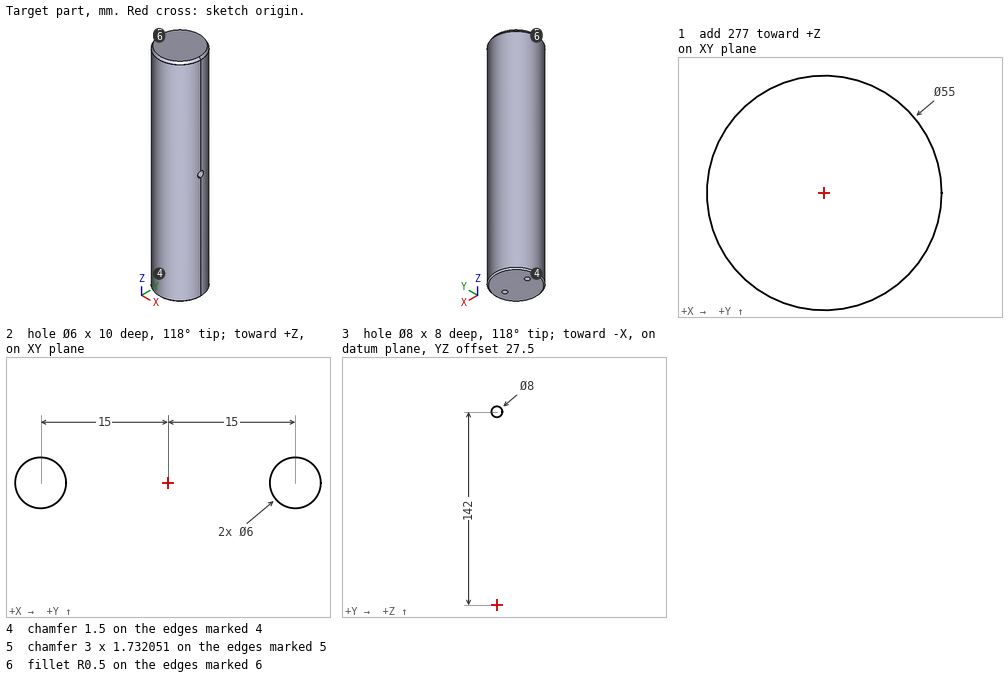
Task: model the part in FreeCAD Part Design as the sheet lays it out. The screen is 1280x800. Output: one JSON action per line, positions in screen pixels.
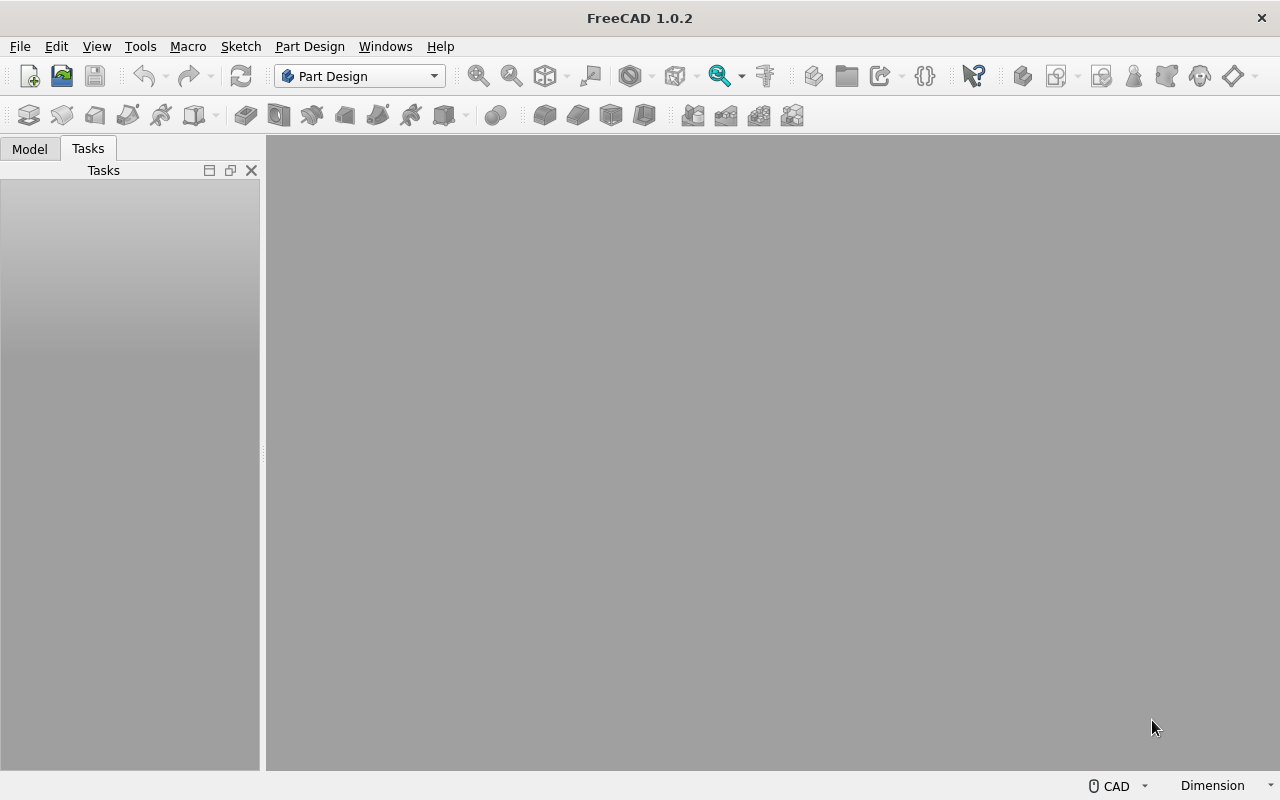
{"action": "left_click", "coordinate": [29, 76]}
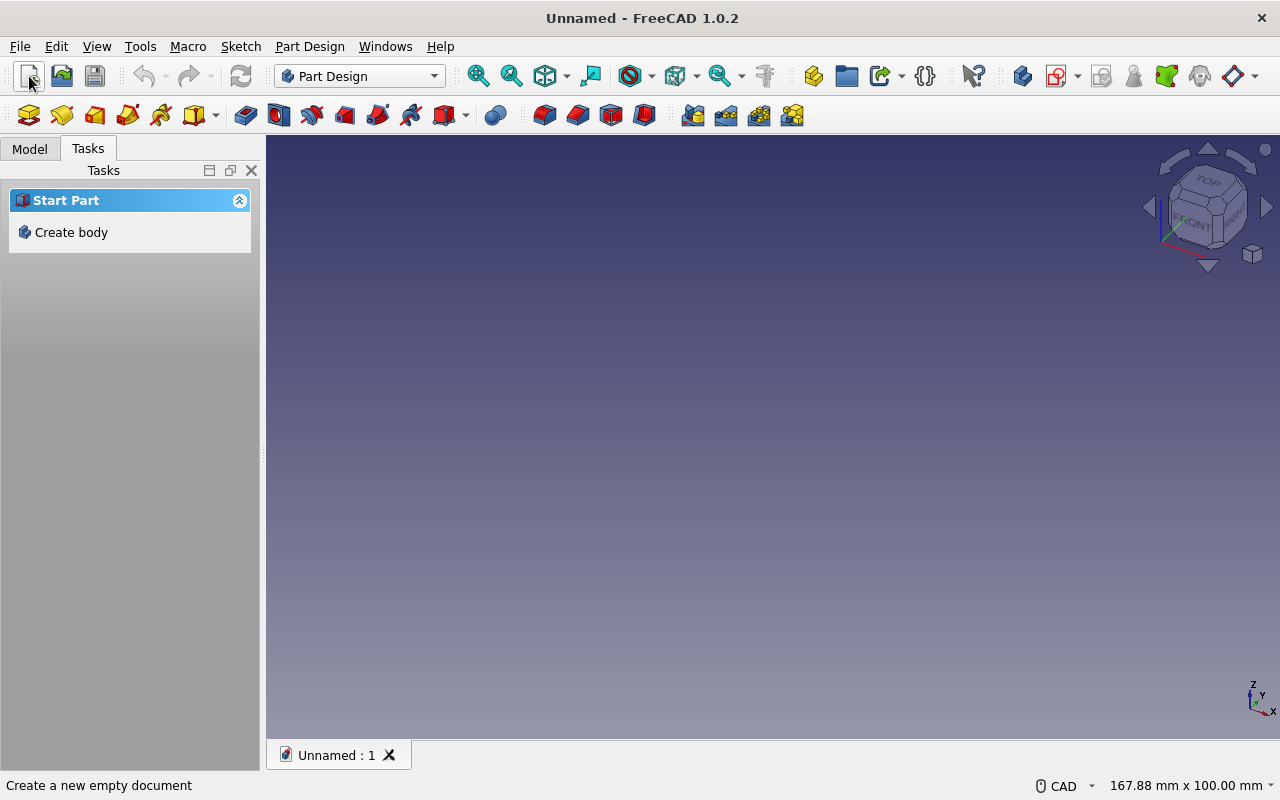
{"action": "left_click", "coordinate": [1056, 76]}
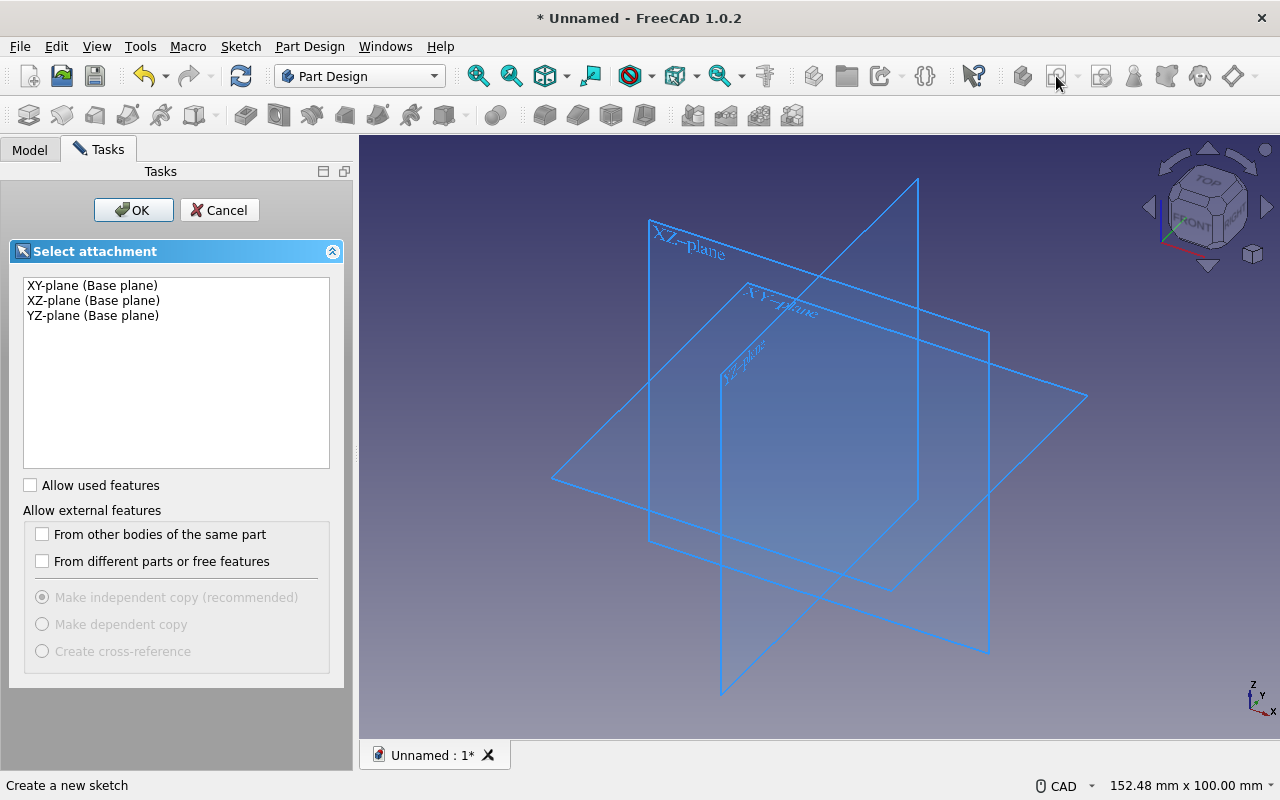
{"action": "left_click", "coordinate": [84, 286]}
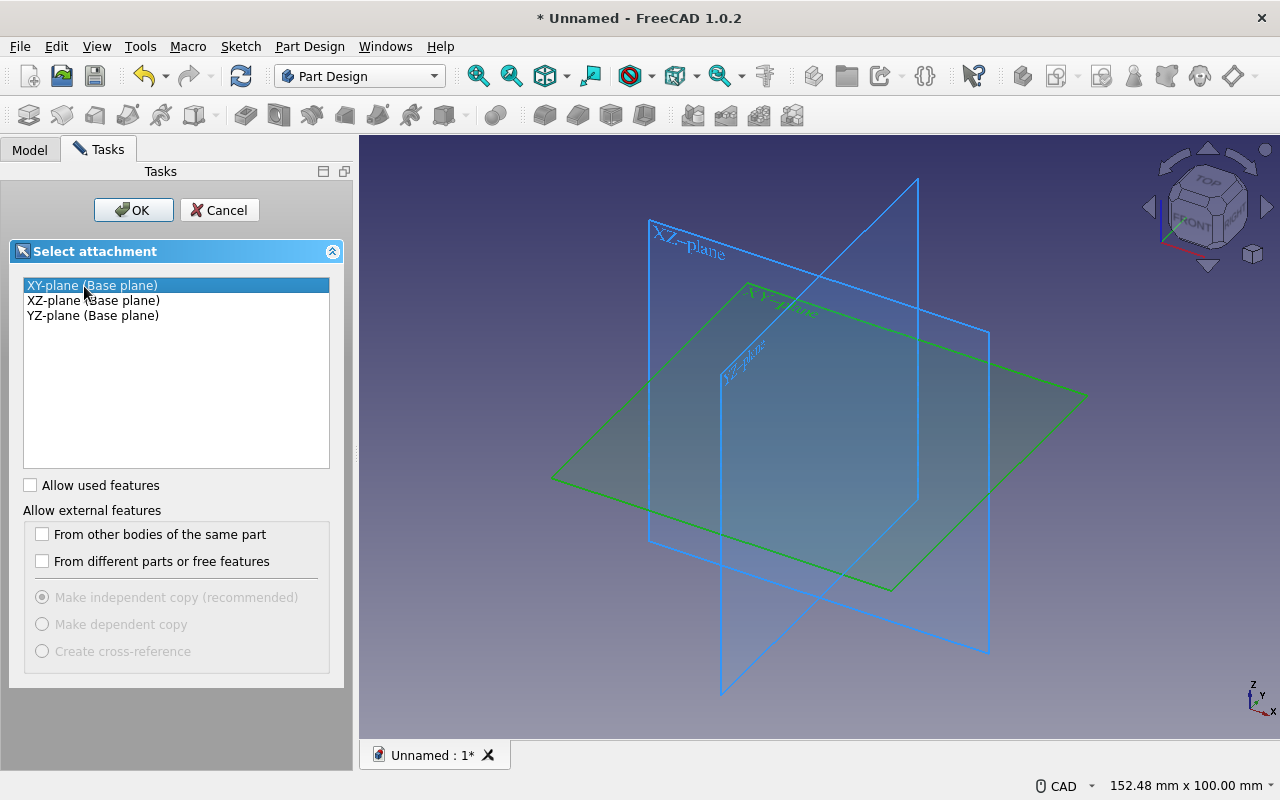
{"action": "left_click", "coordinate": [134, 210]}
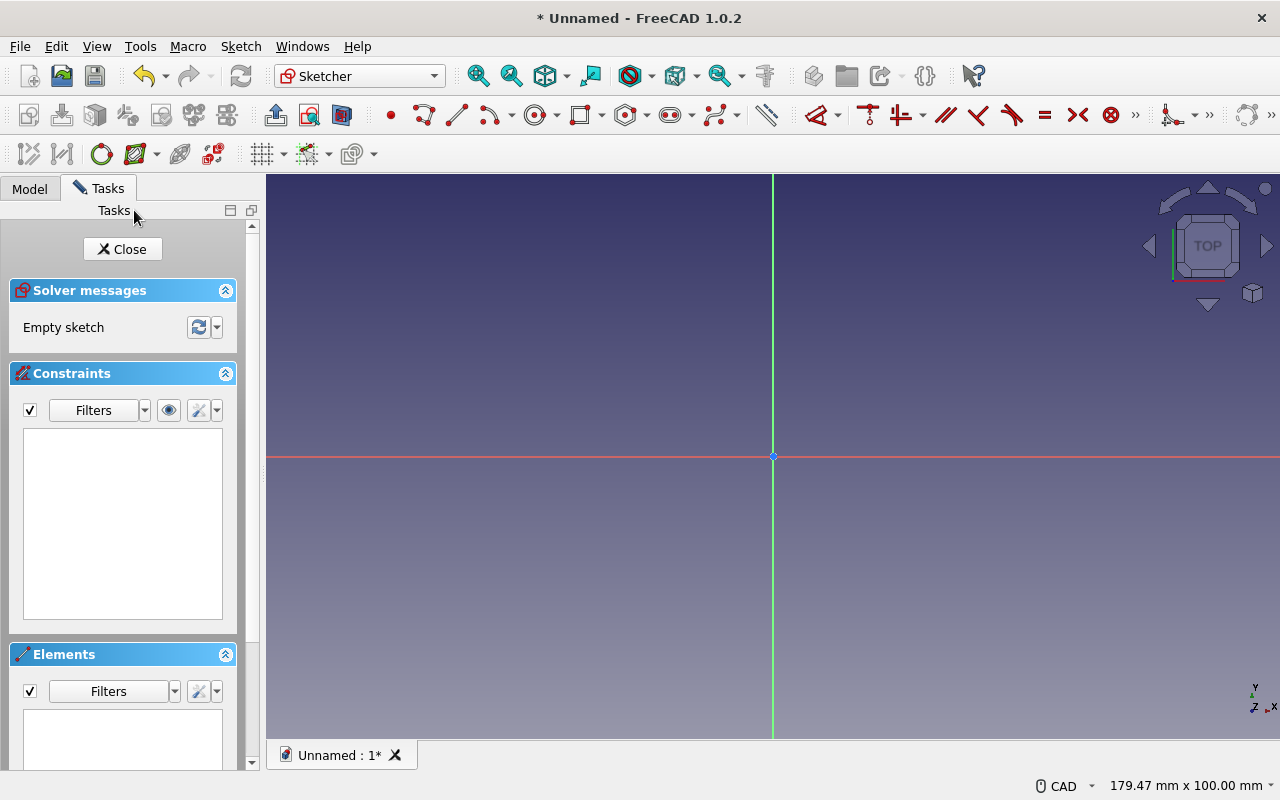
{"action": "left_click", "coordinate": [534, 116]}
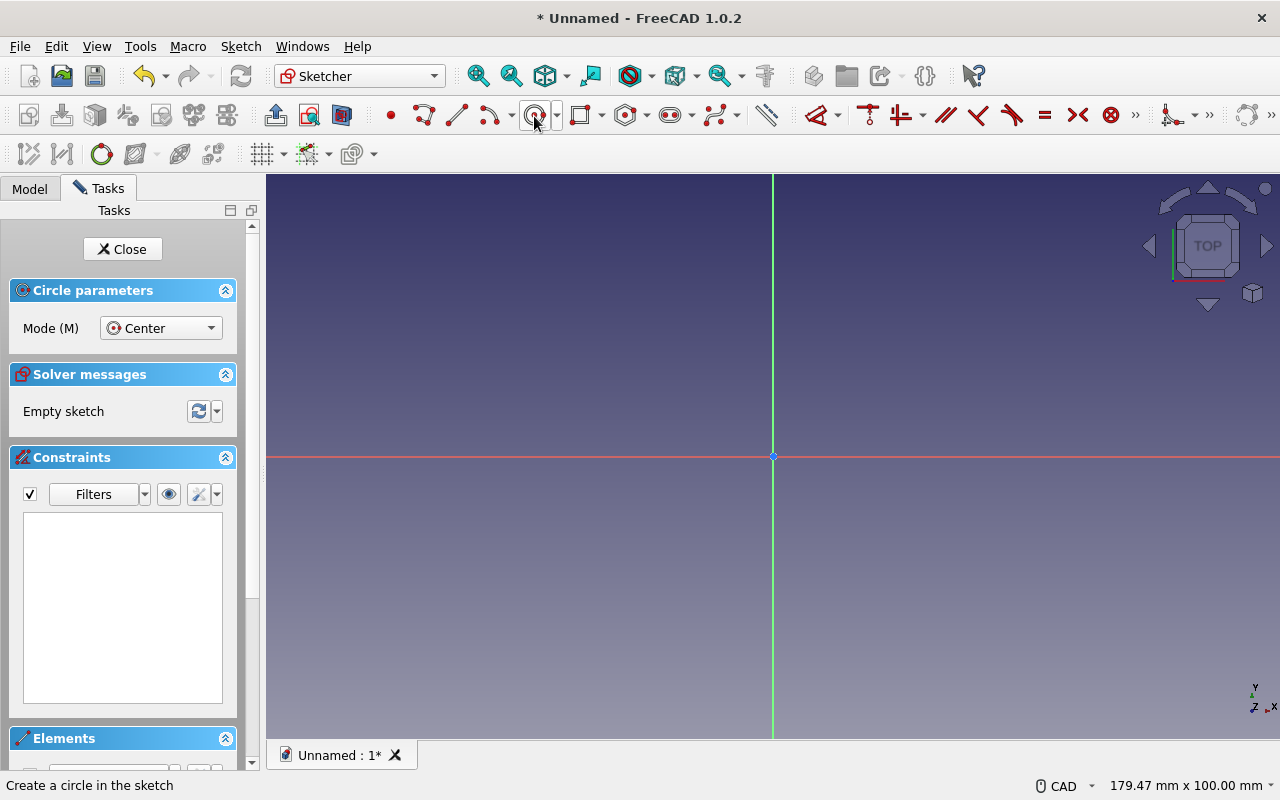
{"action": "left_click", "coordinate": [773, 456]}
{"action": "left_click", "coordinate": [883, 347]}
{"action": "key", "text": "Escape"}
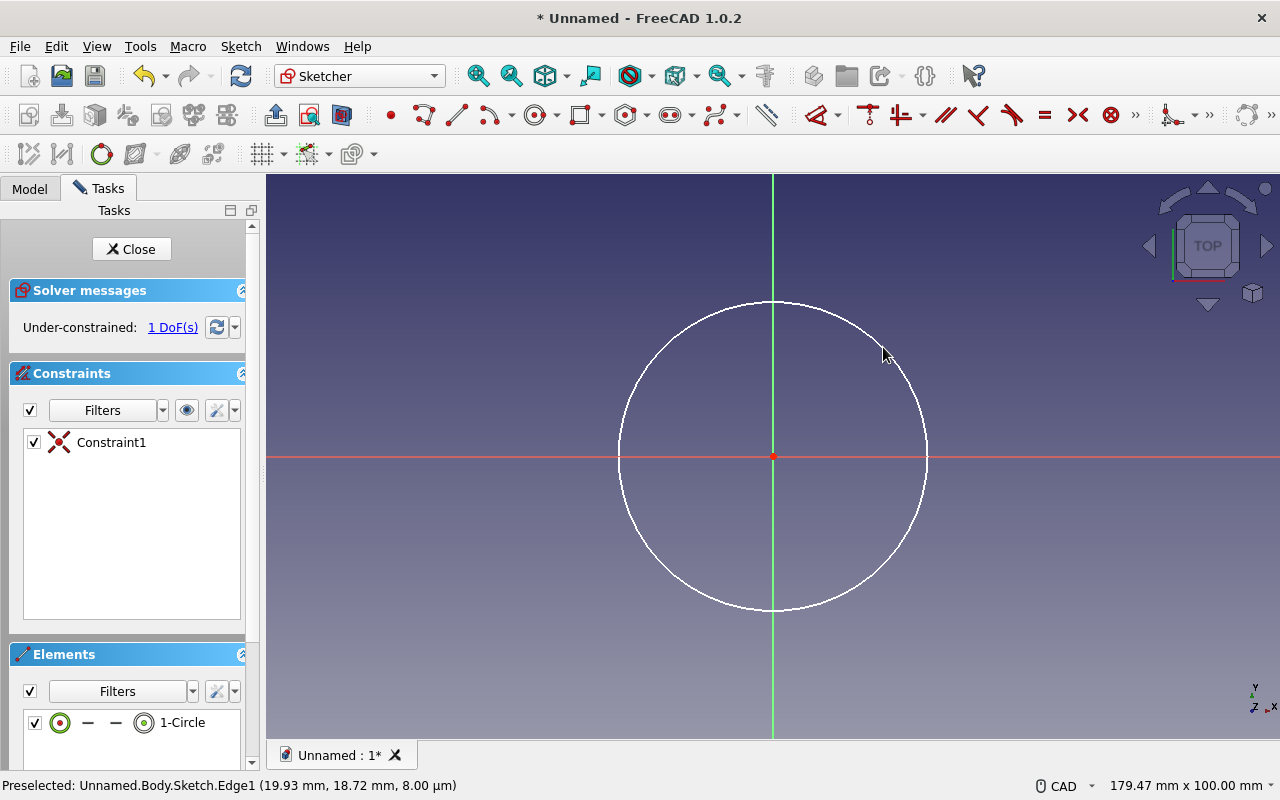
{"action": "key", "text": "d"}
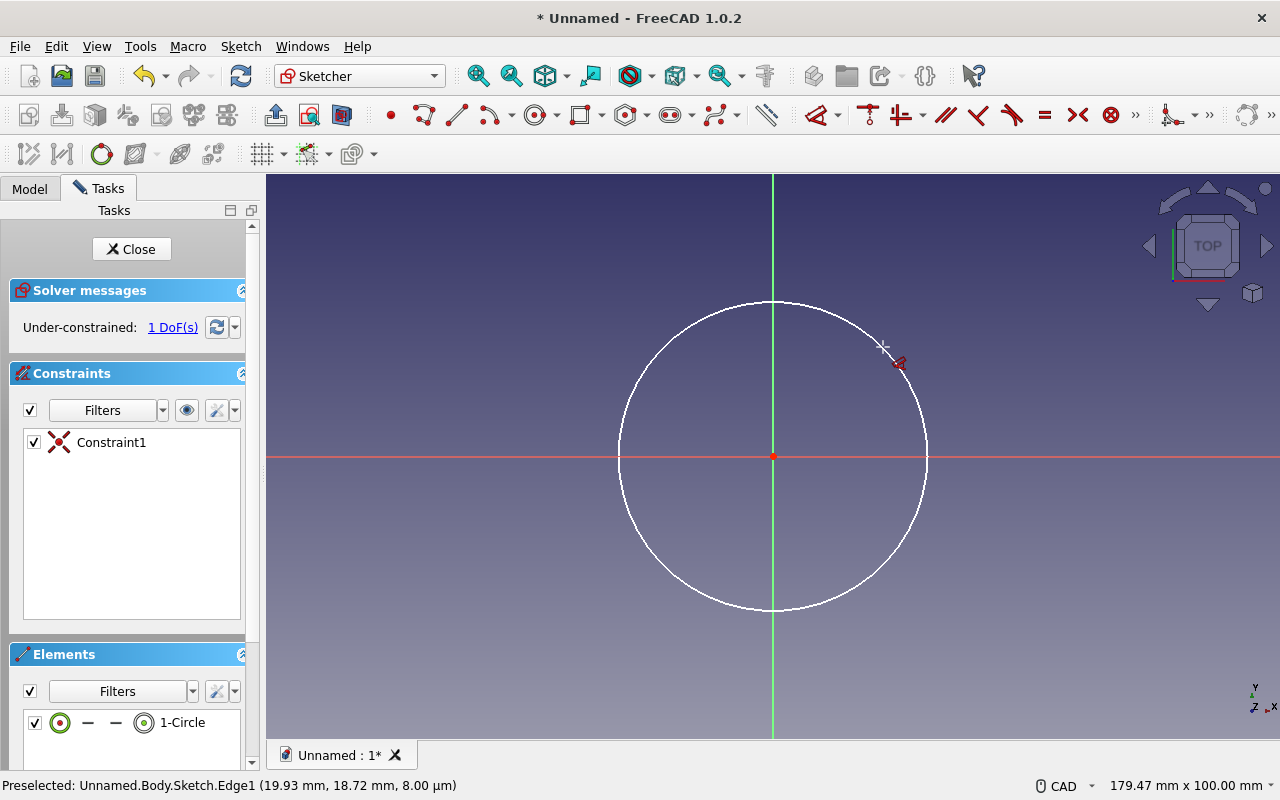
{"action": "left_click", "coordinate": [882, 347]}
{"action": "left_click", "coordinate": [905, 324]}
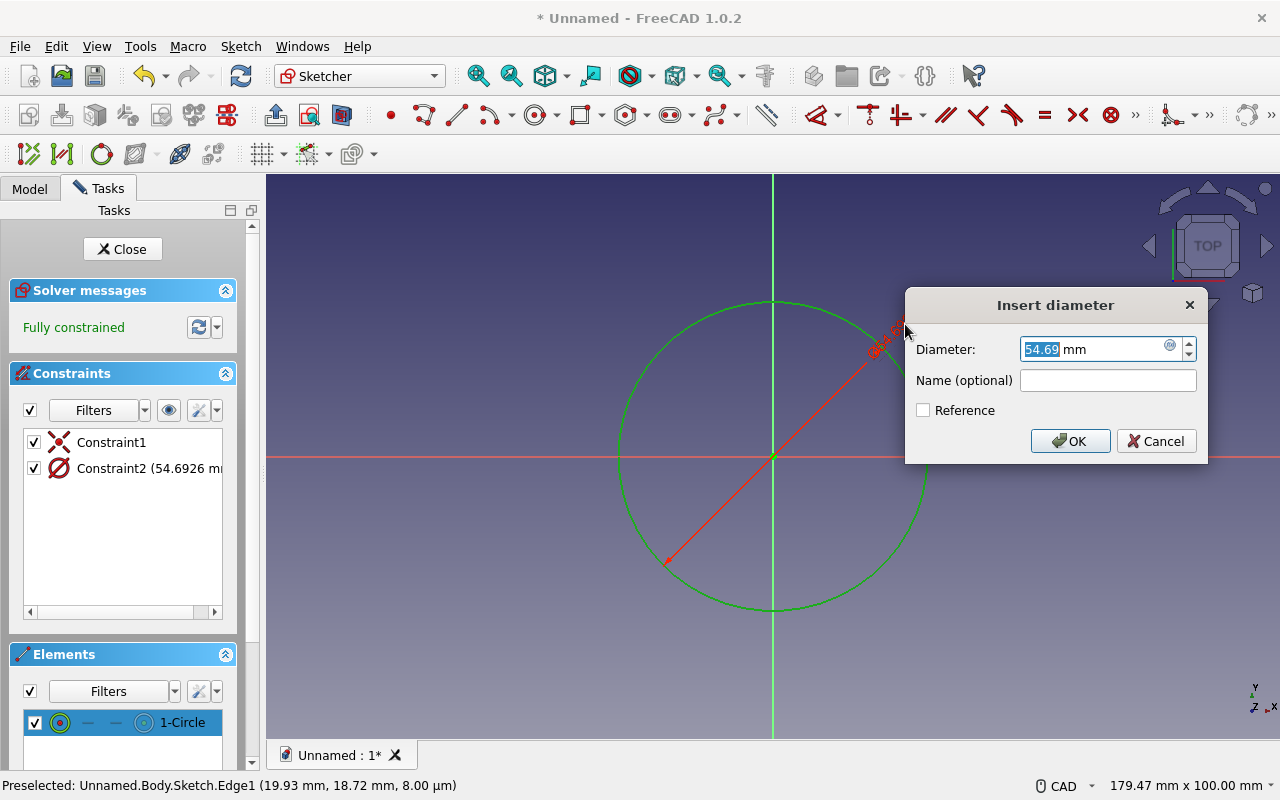
{"action": "type", "text": "55"}
{"action": "key", "text": "Return"}
{"action": "key", "text": "Escape"}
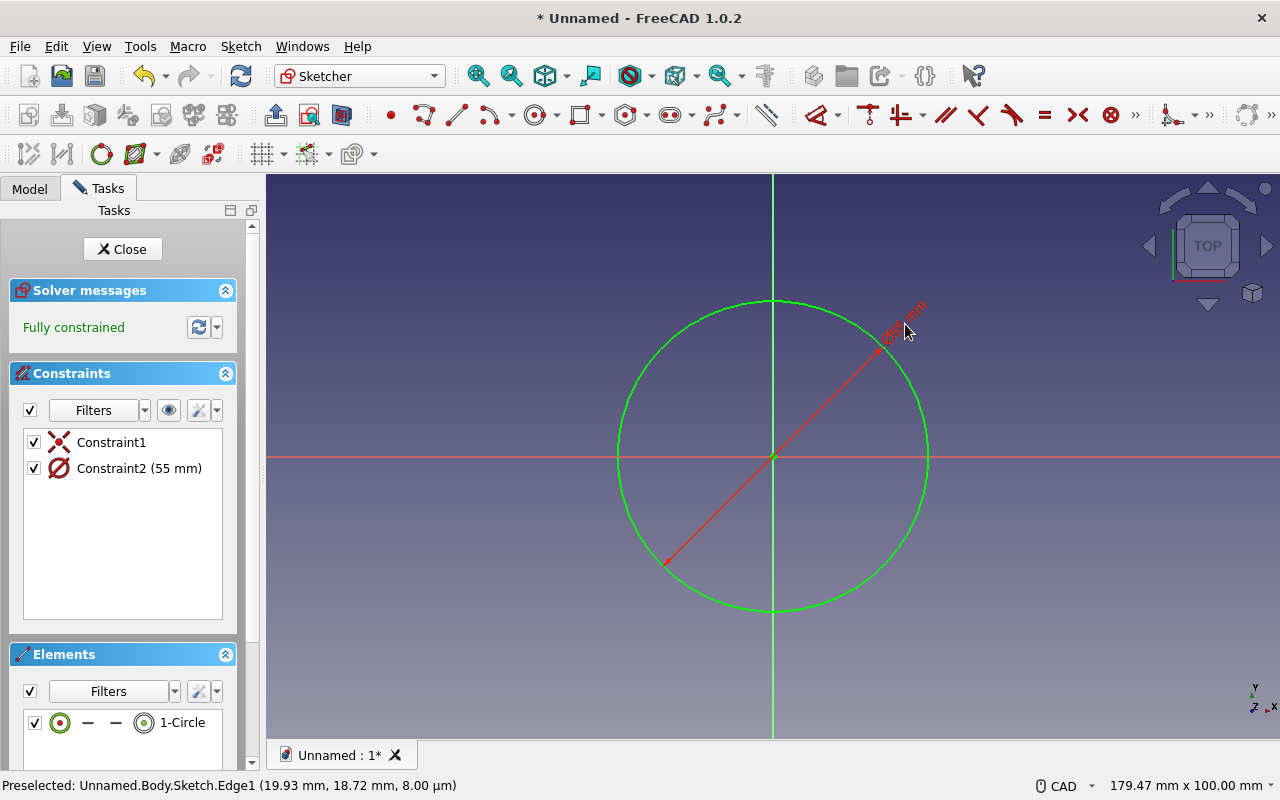
{"action": "left_click", "coordinate": [123, 249]}